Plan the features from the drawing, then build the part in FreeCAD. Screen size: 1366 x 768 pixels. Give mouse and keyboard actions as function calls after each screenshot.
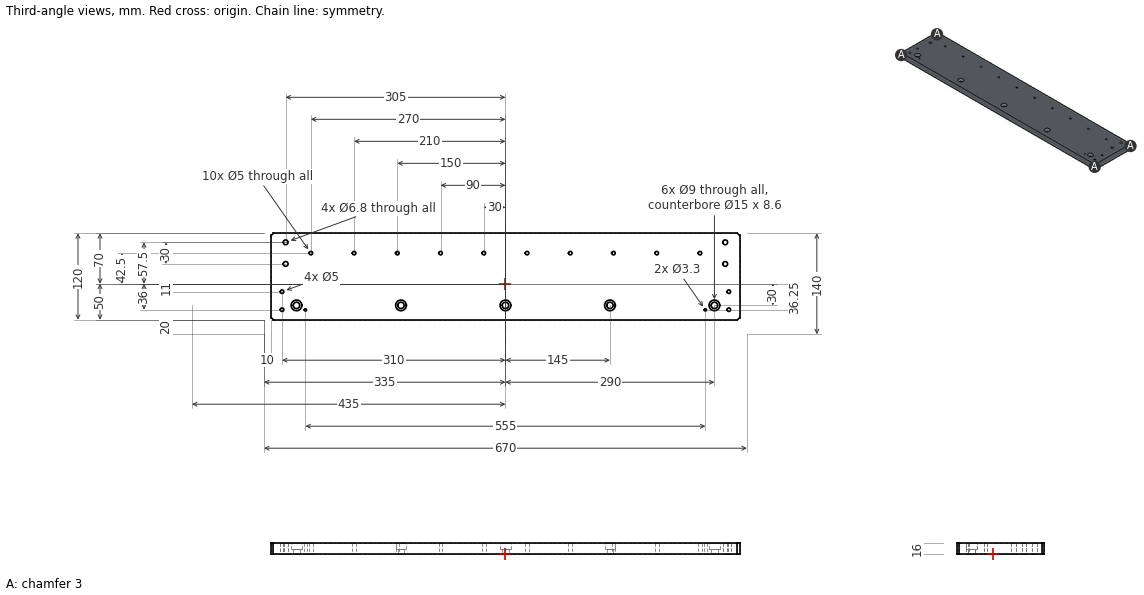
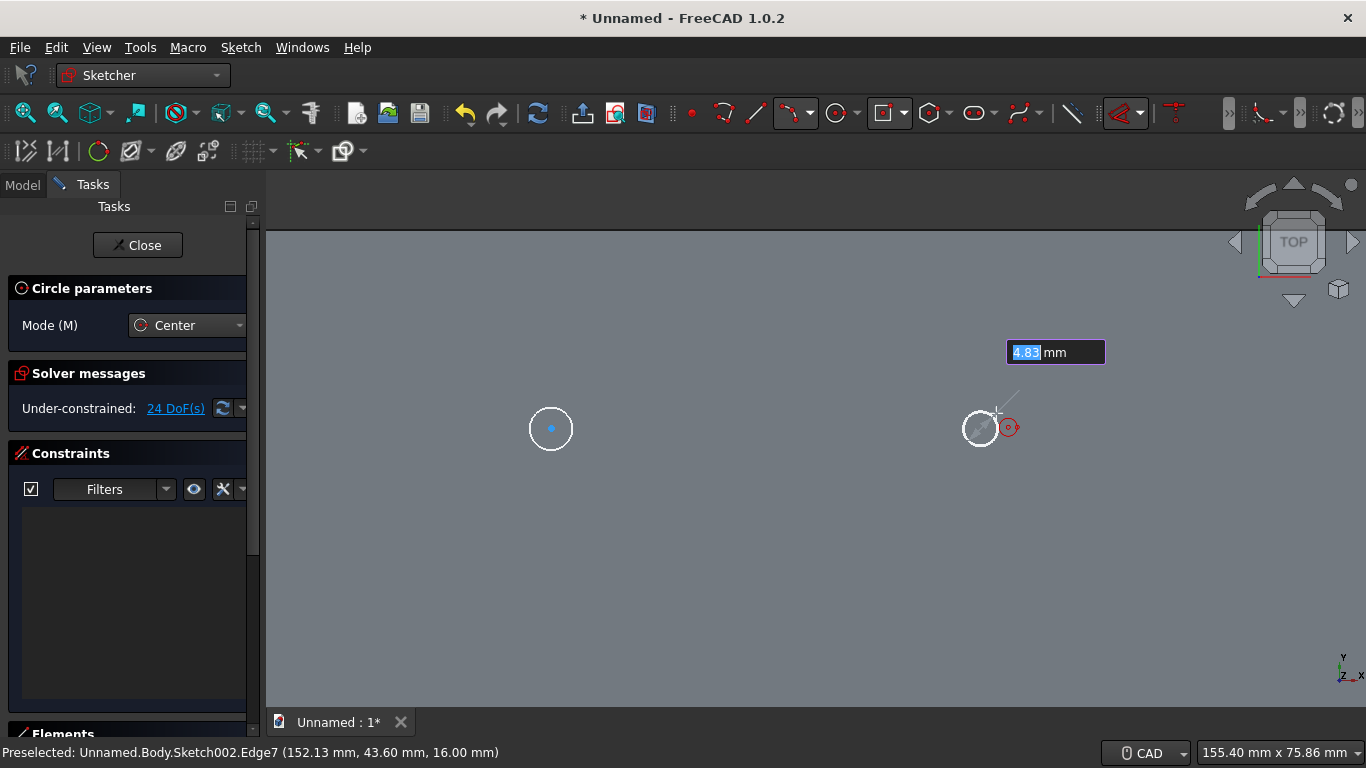
click(990, 412)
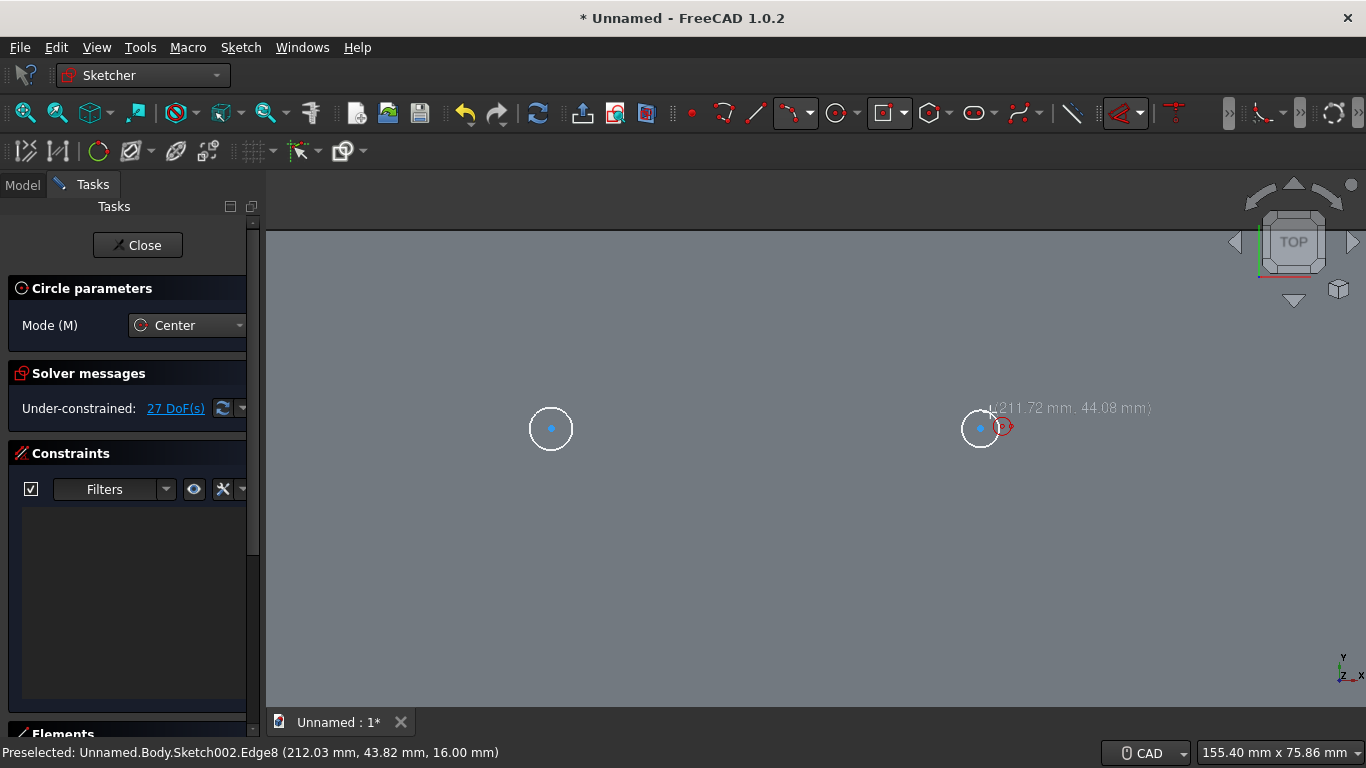
scroll(996, 413, down, 9)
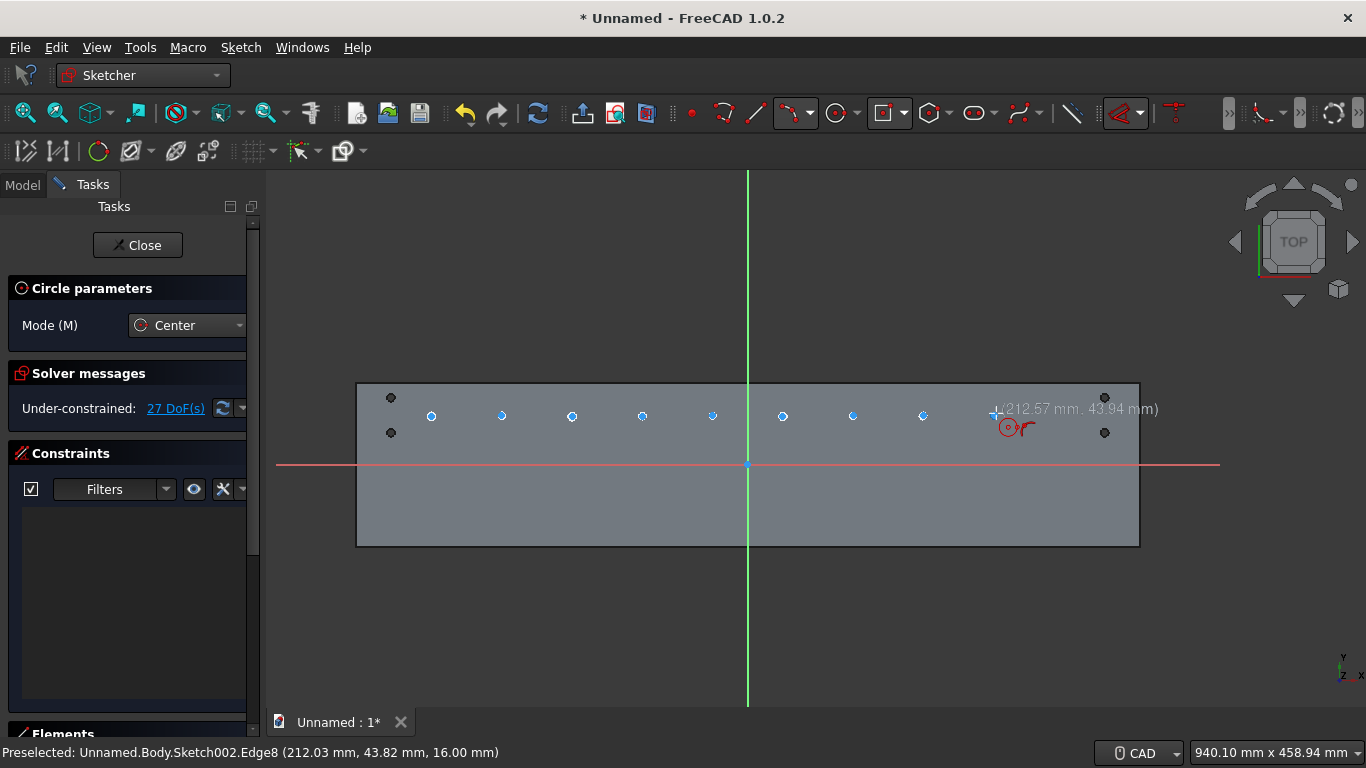
scroll(1064, 415, up, 11)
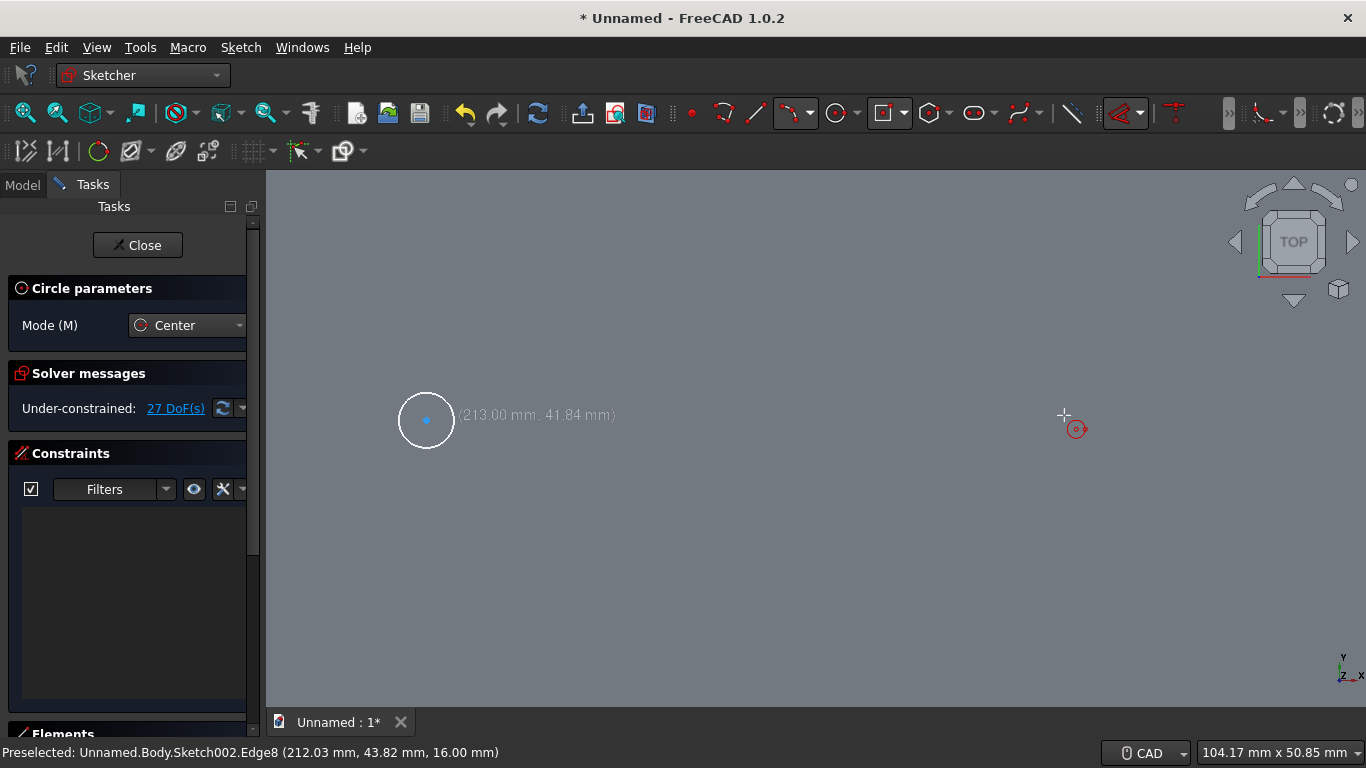
scroll(1064, 415, down, 11)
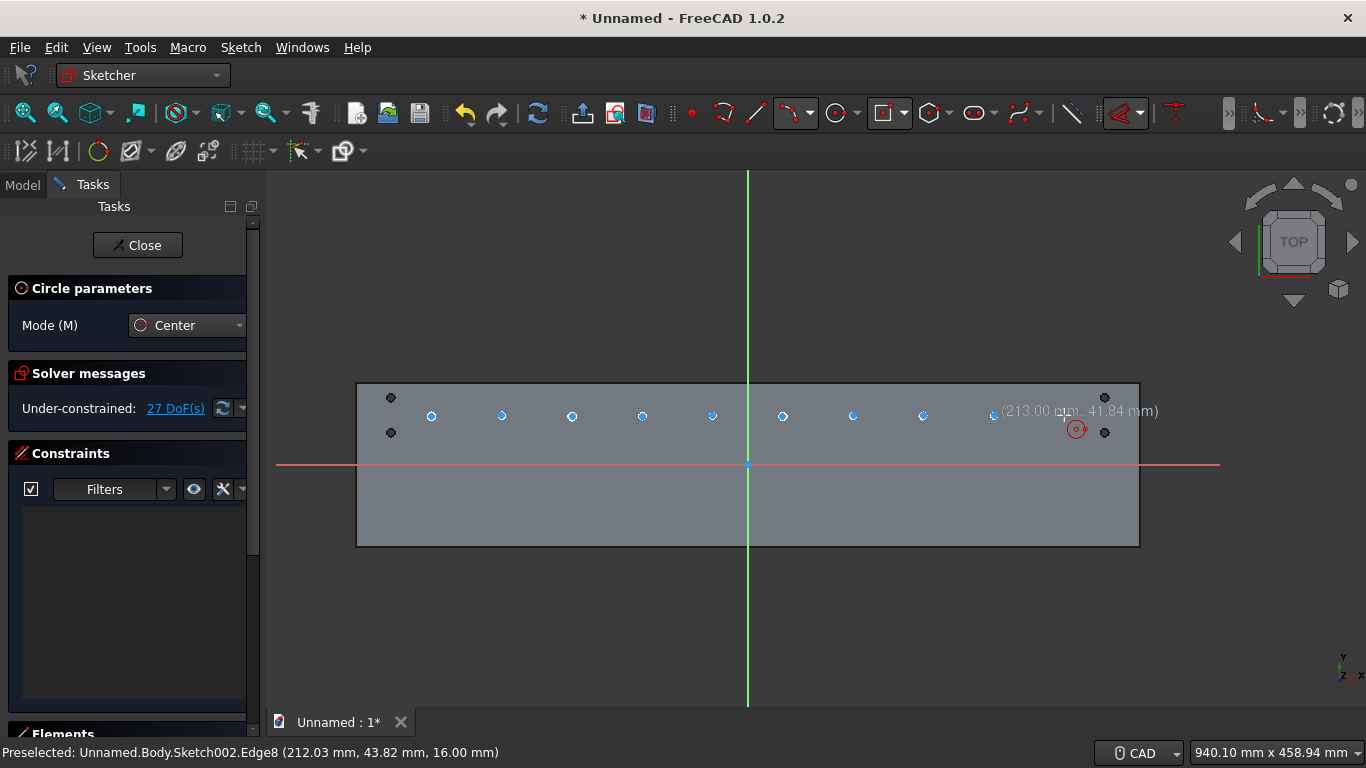
click(1064, 415)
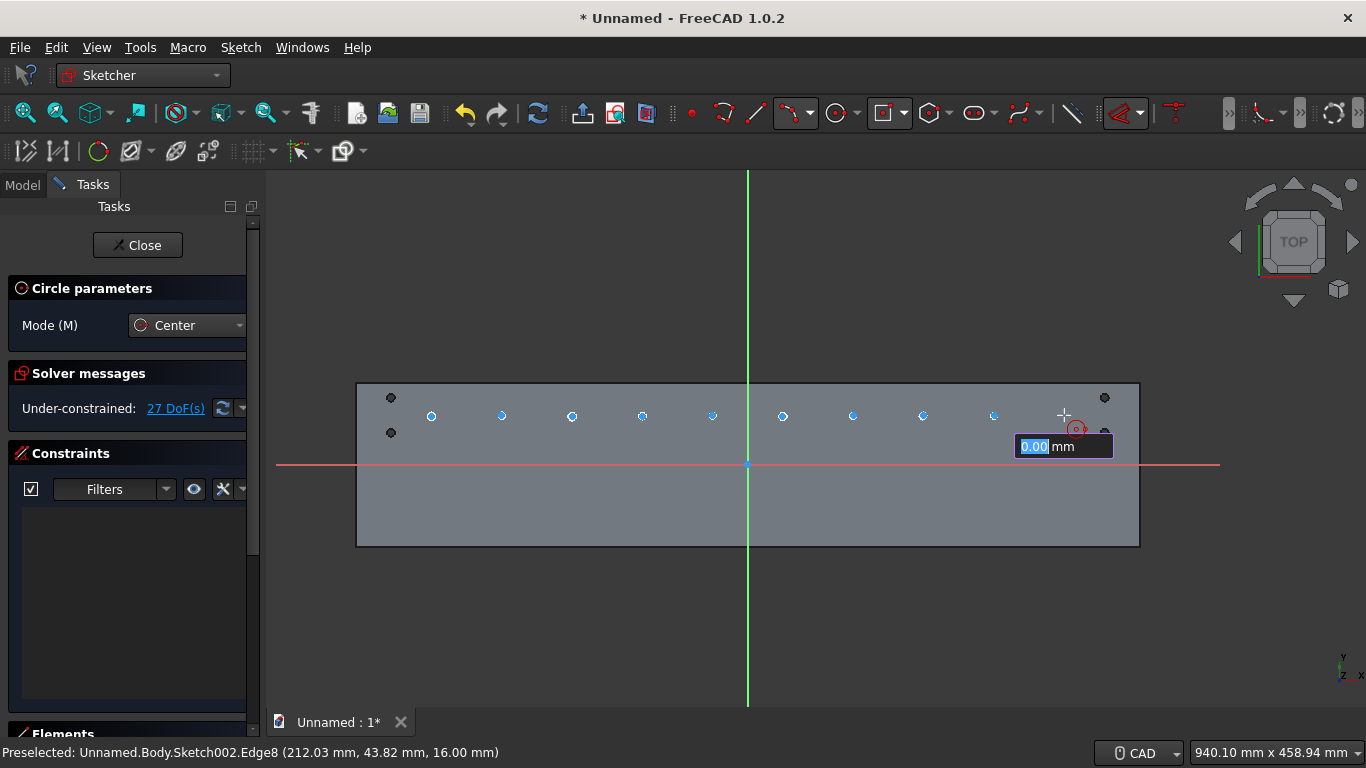
scroll(1066, 413, up, 9)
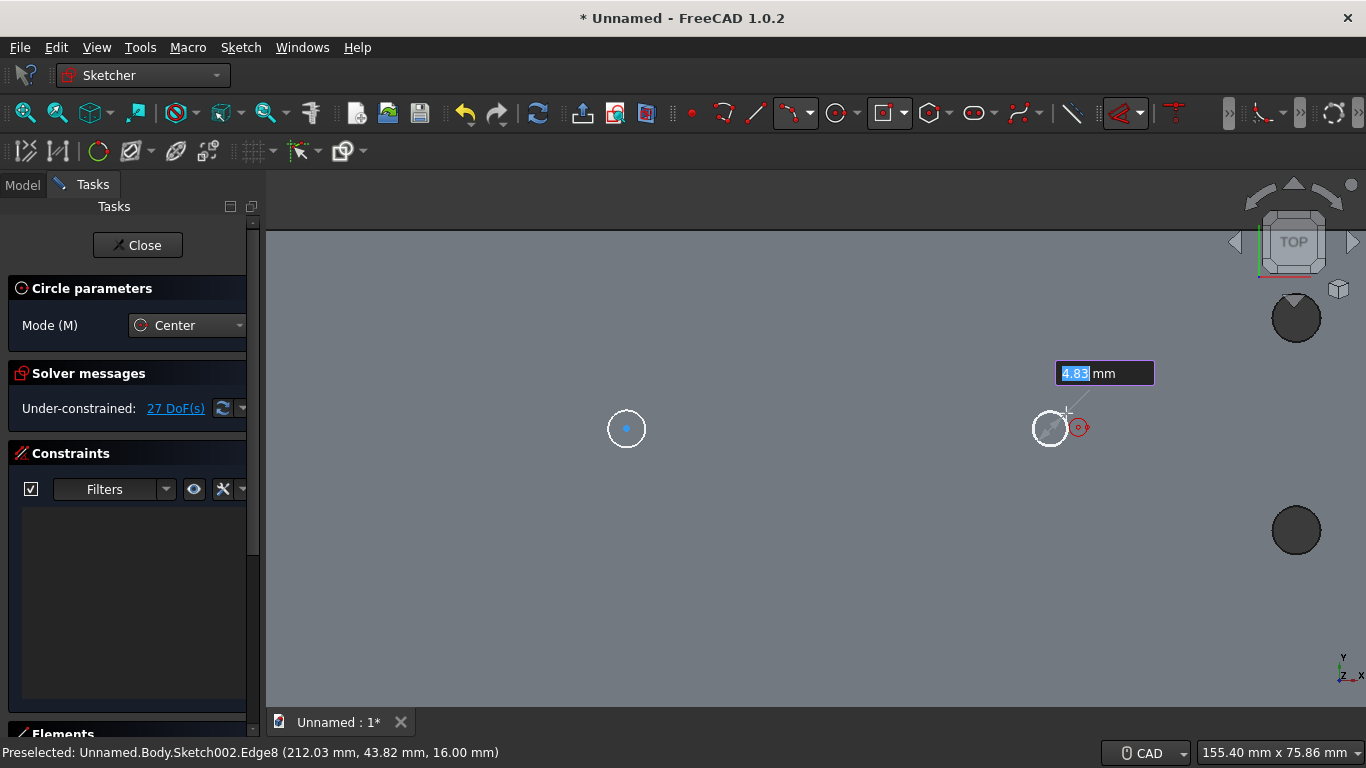
click(1061, 412)
key(Escape)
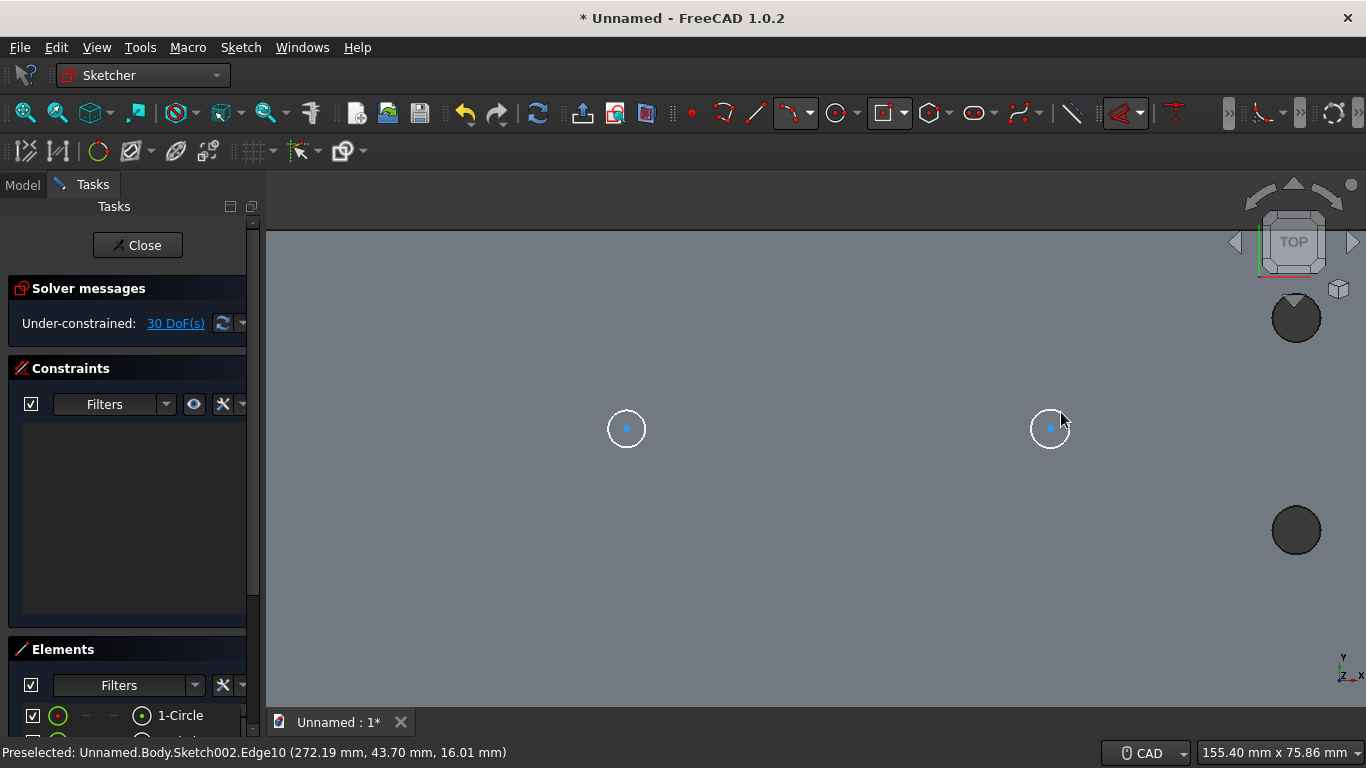
scroll(1066, 413, down, 9)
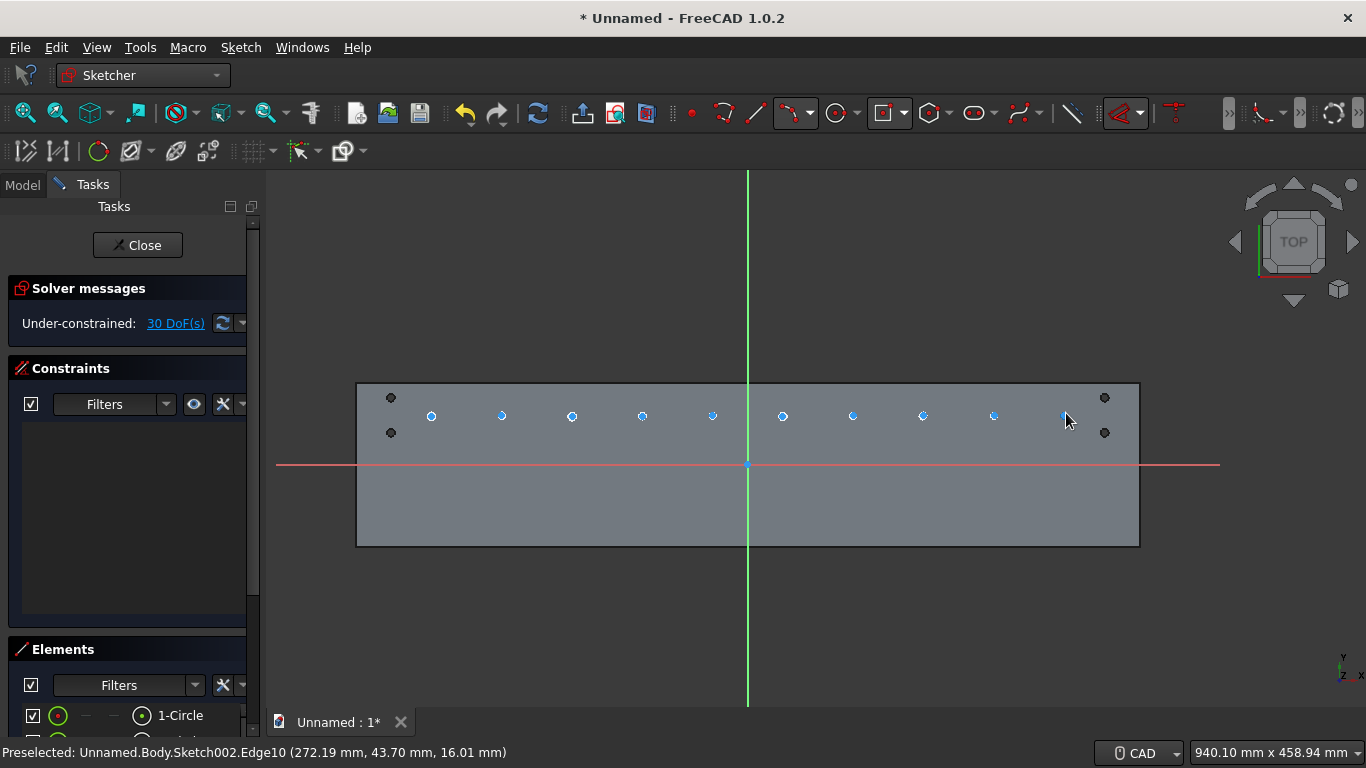
scroll(434, 414, up, 7)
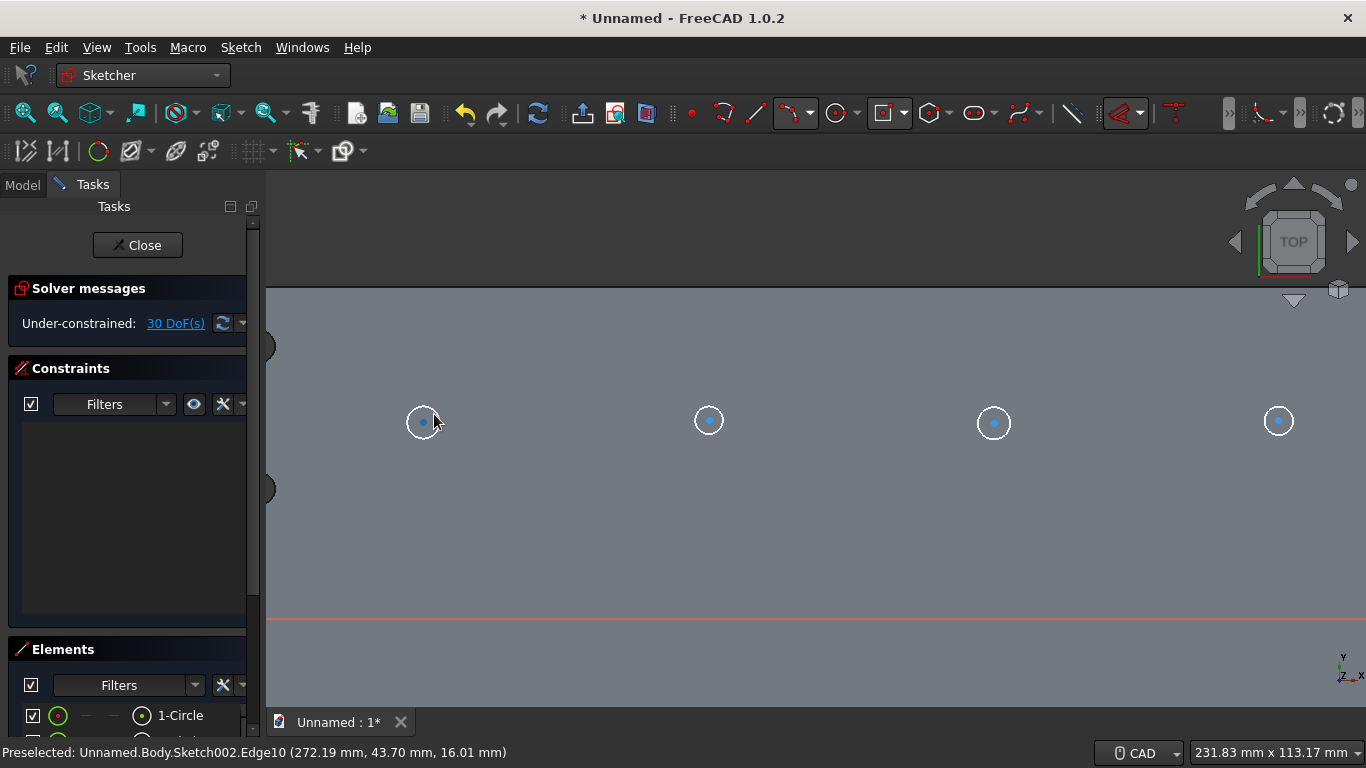
click(435, 411)